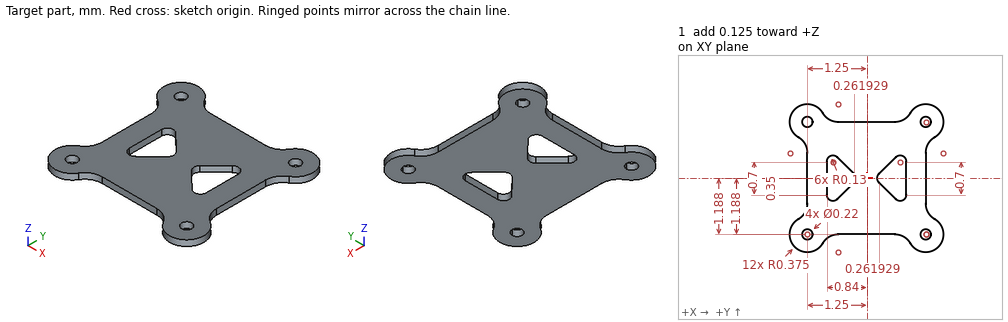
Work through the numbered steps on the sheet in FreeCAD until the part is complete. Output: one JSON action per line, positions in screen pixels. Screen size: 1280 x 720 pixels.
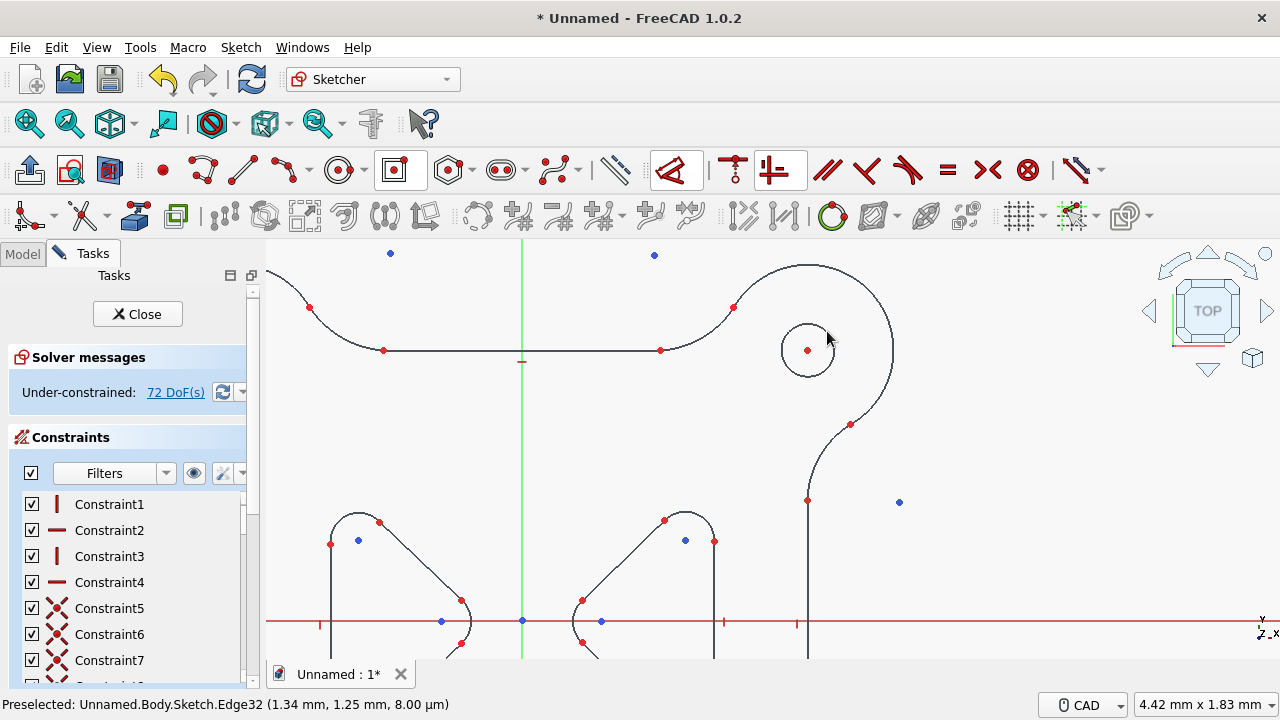
{"action": "scroll", "coordinate": [811, 349], "scroll_direction": "down", "scroll_amount": 5}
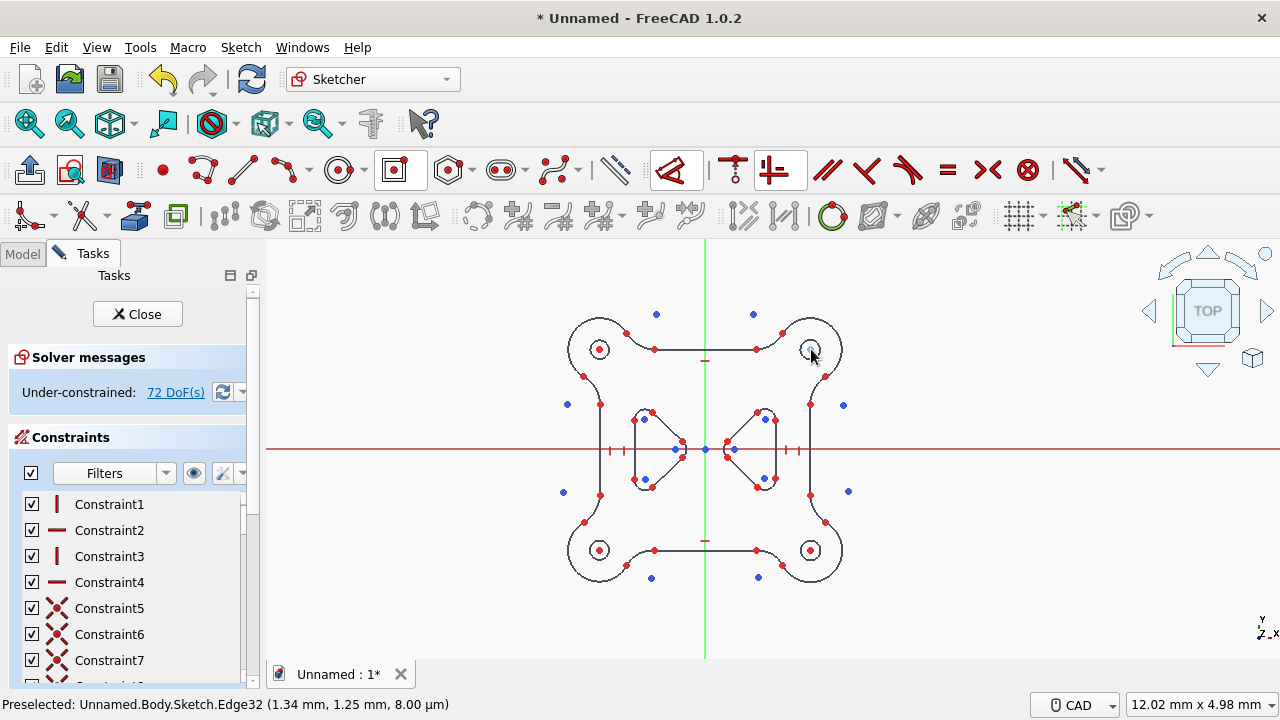
{"action": "left_click", "coordinate": [600, 432]}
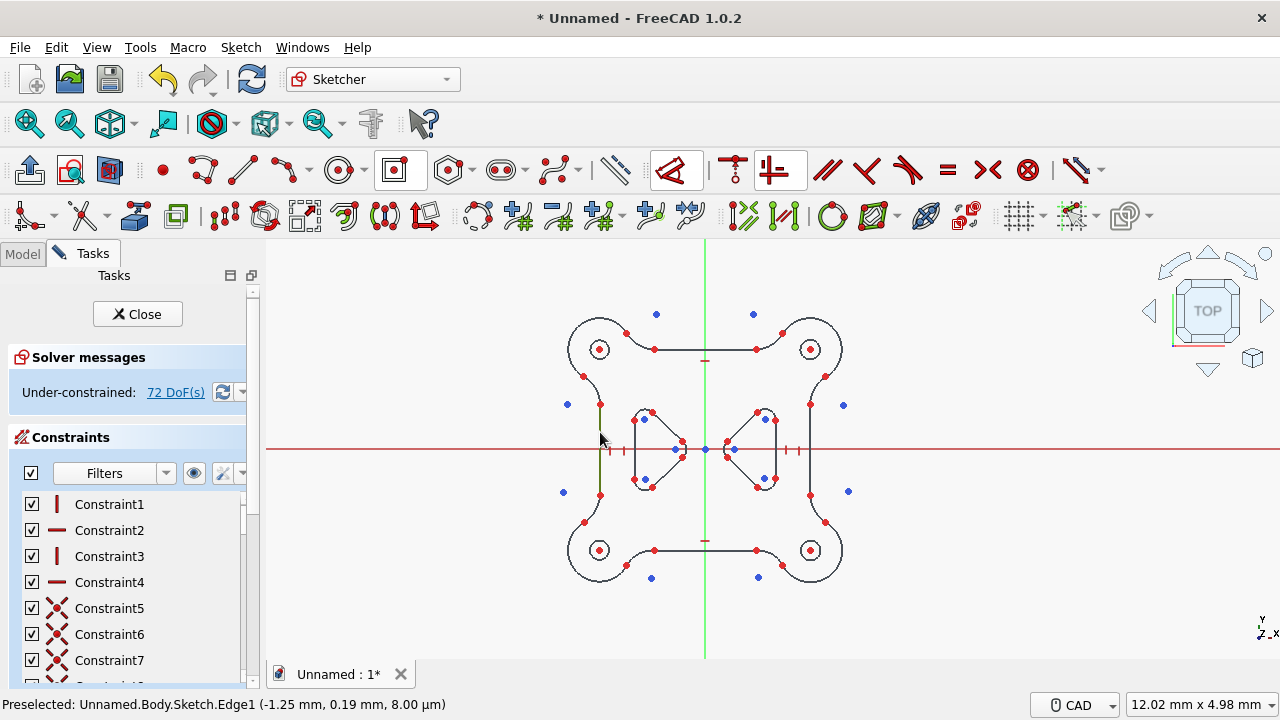
{"action": "scroll", "coordinate": [591, 516], "scroll_direction": "up", "scroll_amount": 2}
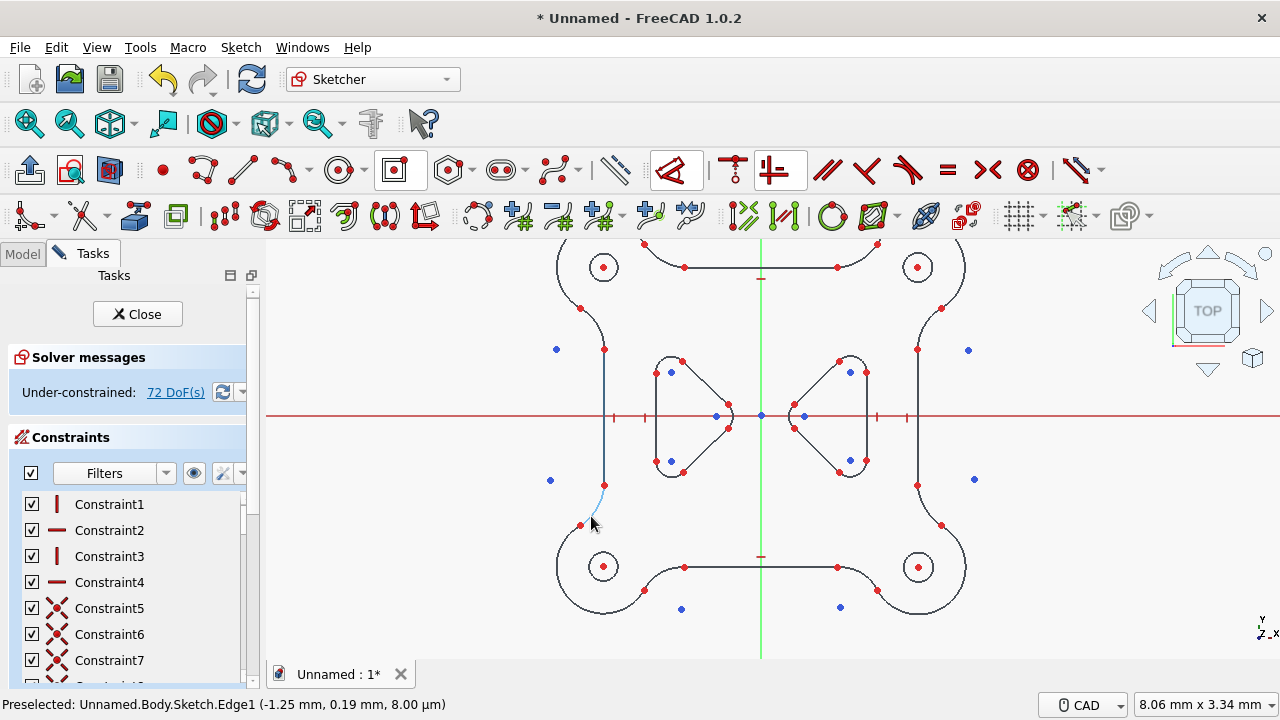
{"action": "left_click", "coordinate": [591, 516]}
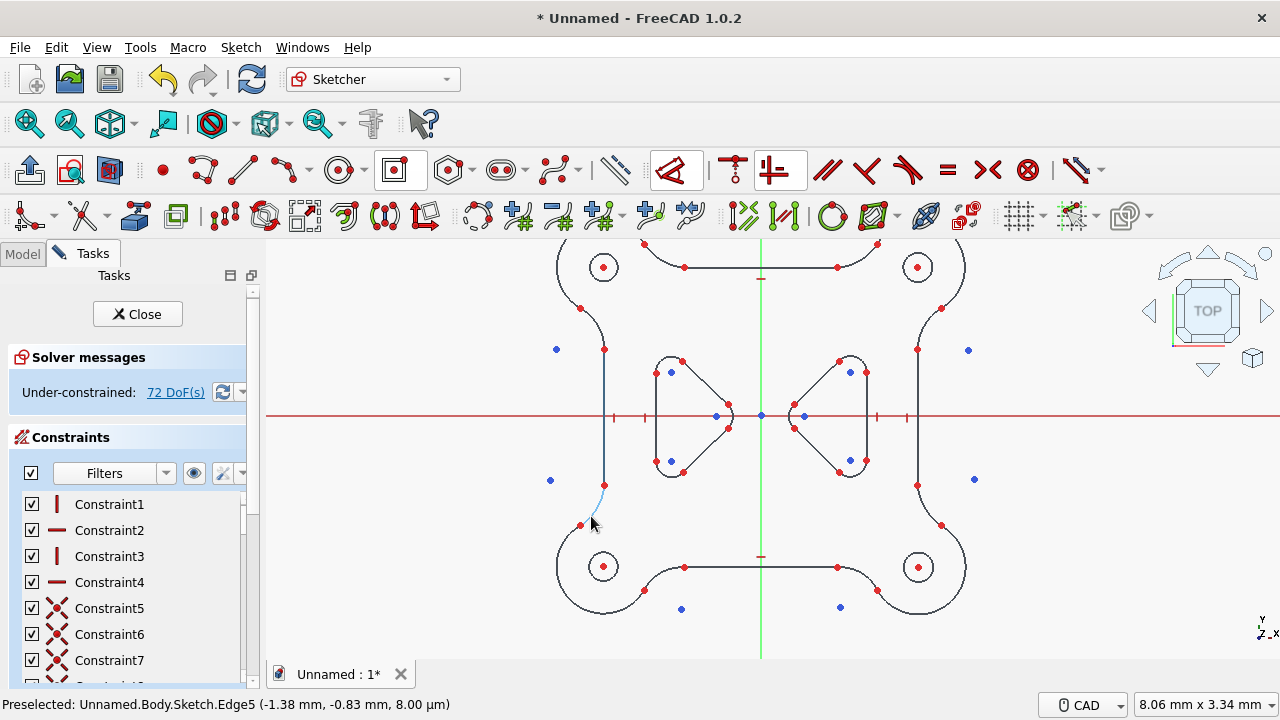
{"action": "left_click", "coordinate": [908, 170]}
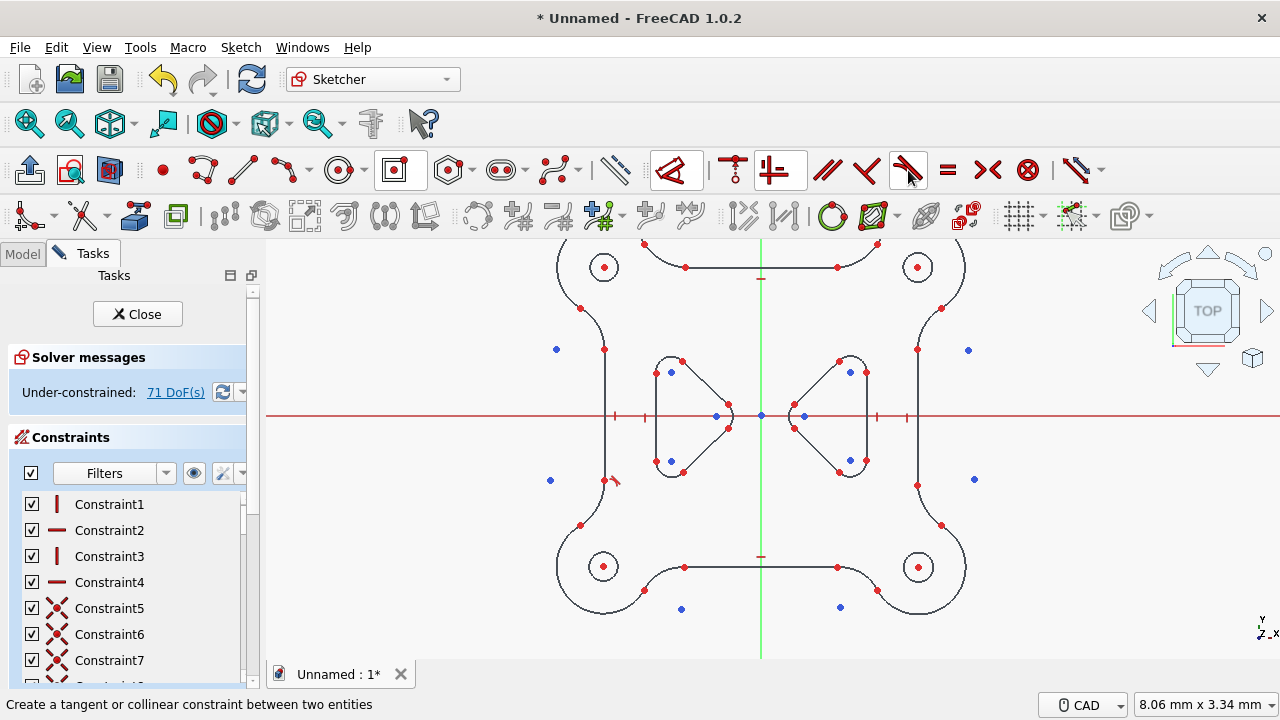
{"action": "left_click", "coordinate": [605, 389]}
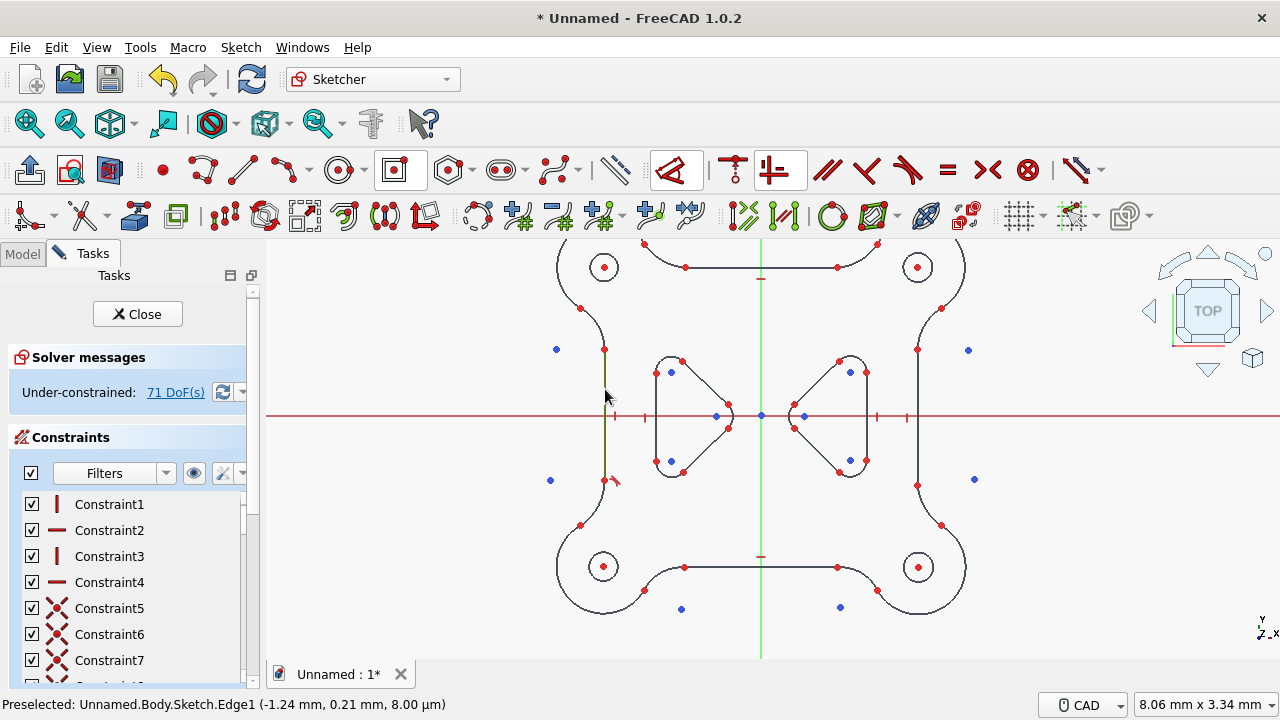
{"action": "left_click", "coordinate": [602, 335]}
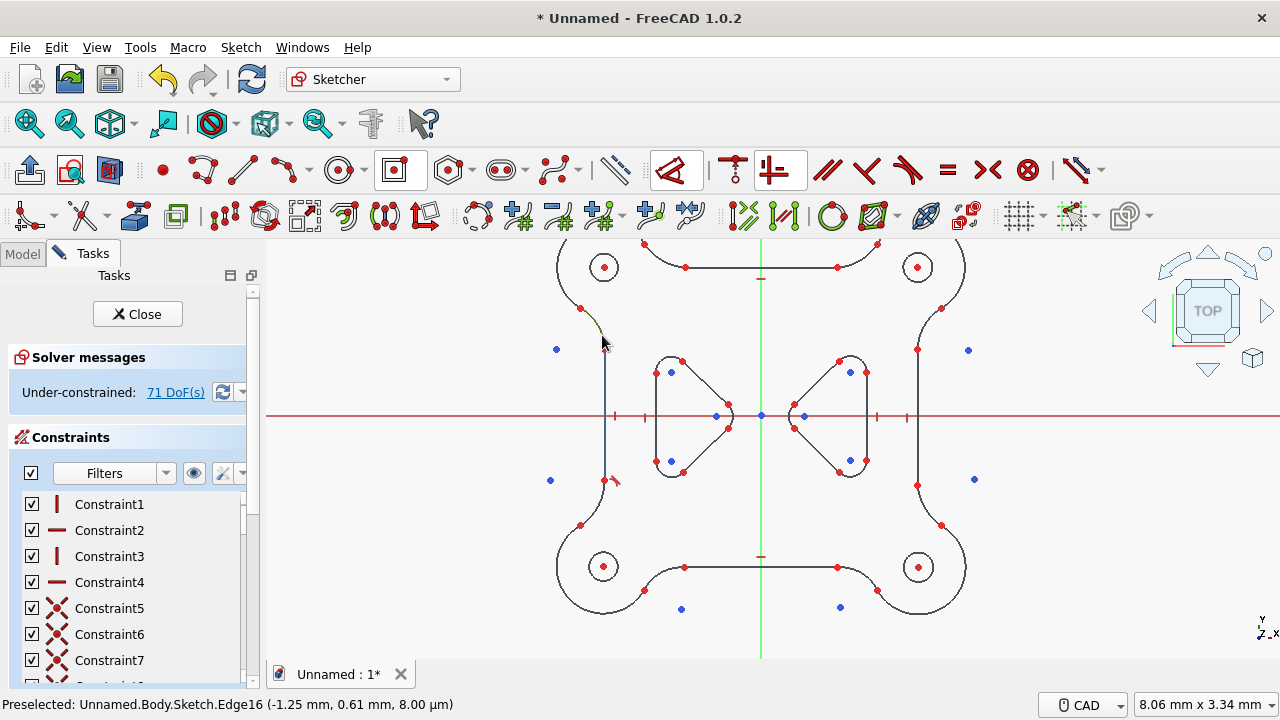
{"action": "left_click", "coordinate": [908, 170]}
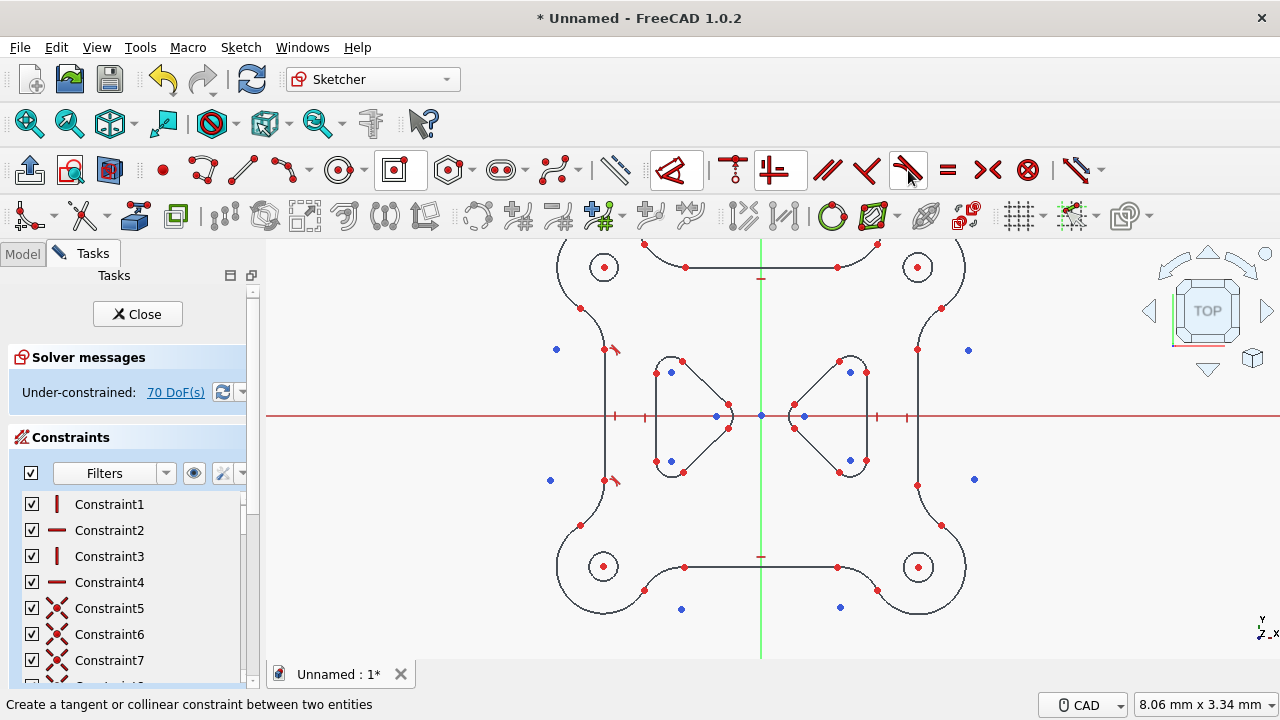
{"action": "left_click", "coordinate": [731, 567]}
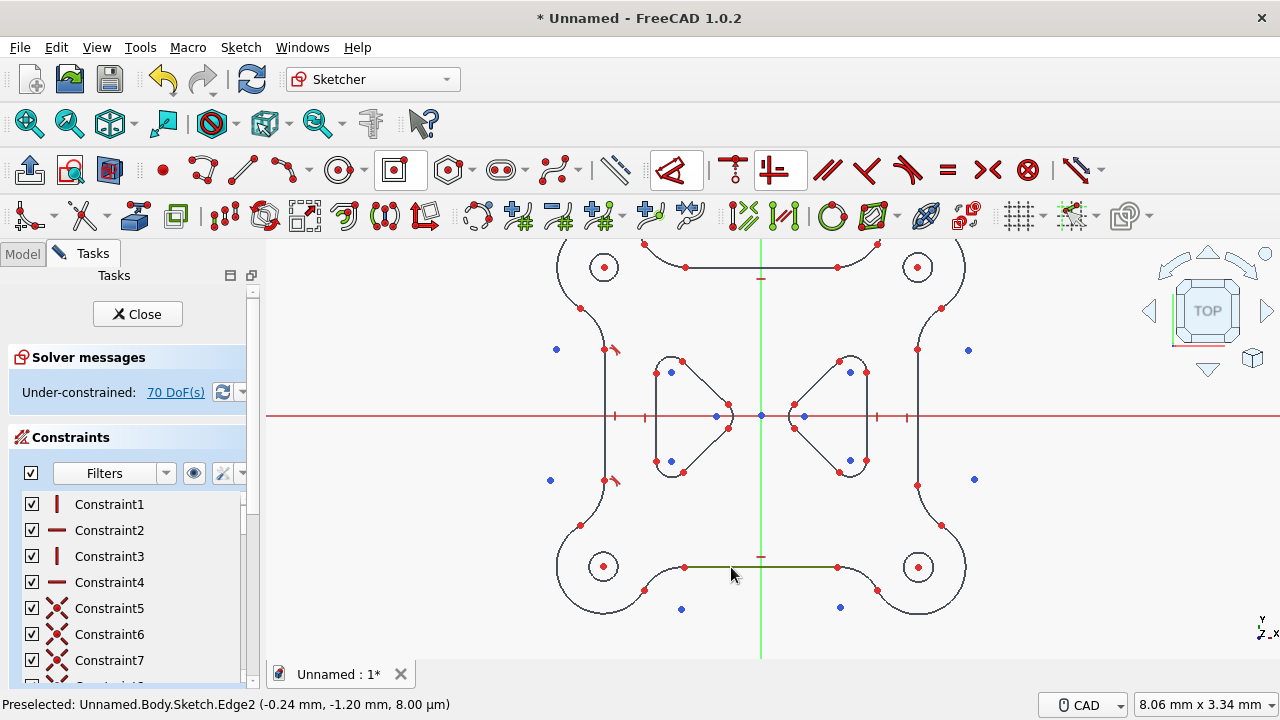
{"action": "left_click", "coordinate": [670, 569]}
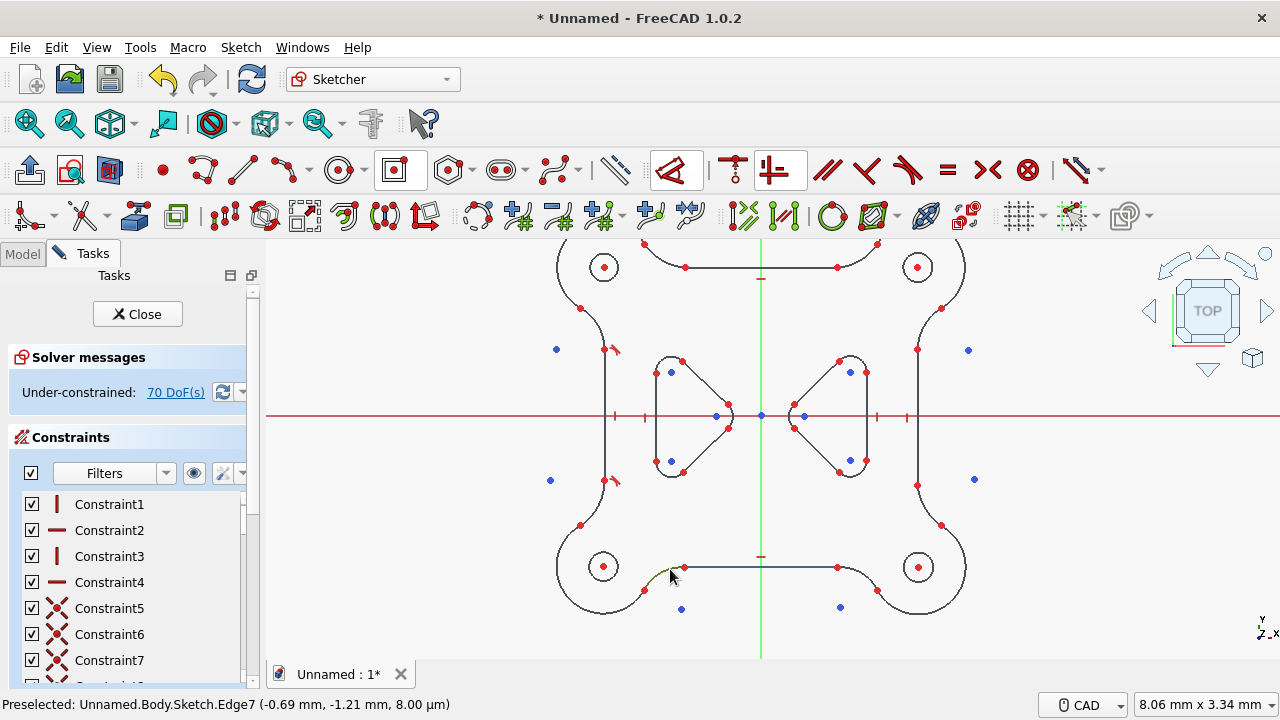
{"action": "left_click", "coordinate": [908, 170]}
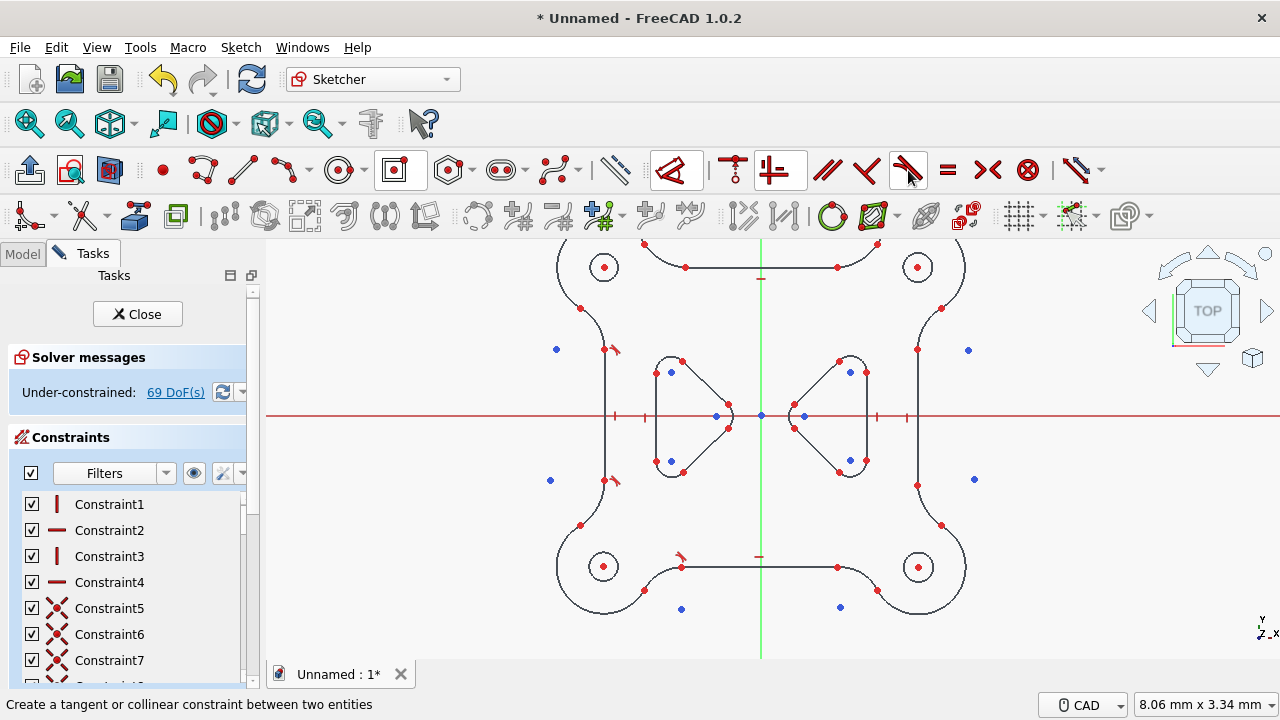
{"action": "left_click", "coordinate": [728, 567]}